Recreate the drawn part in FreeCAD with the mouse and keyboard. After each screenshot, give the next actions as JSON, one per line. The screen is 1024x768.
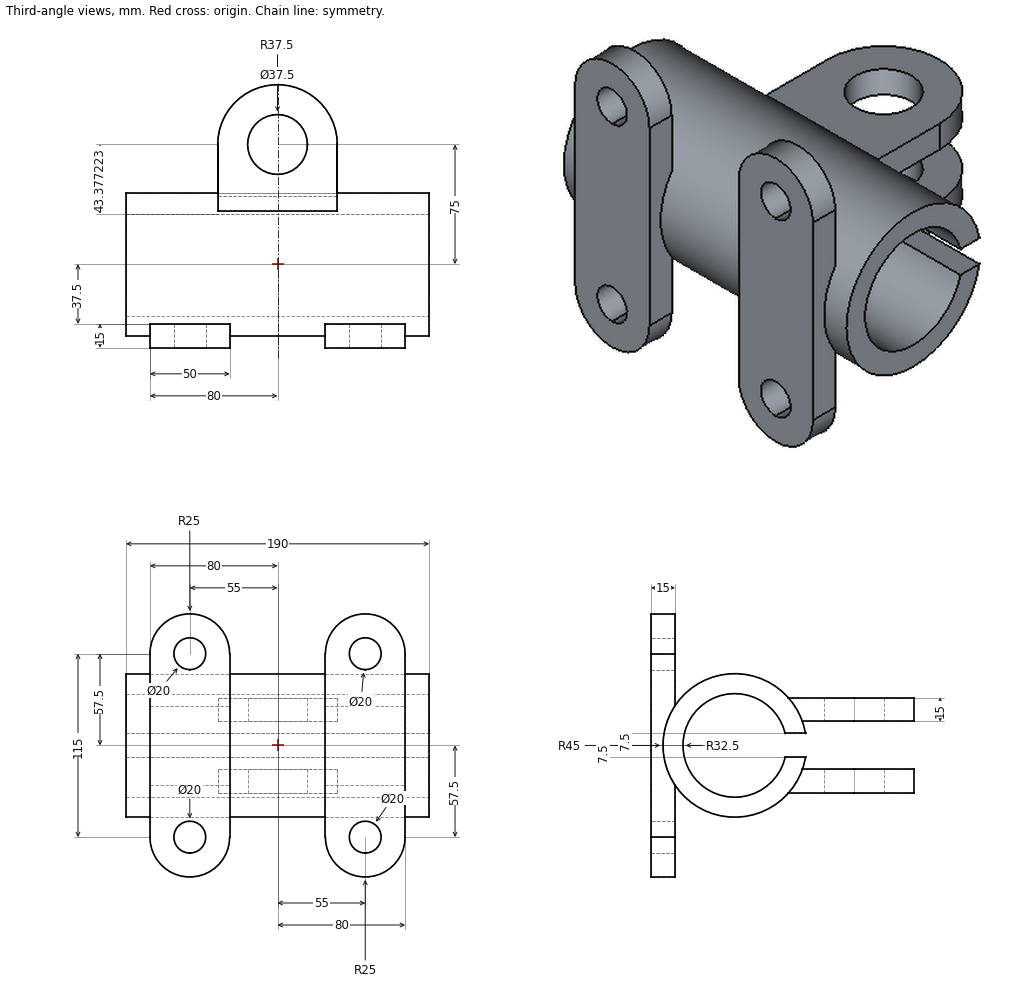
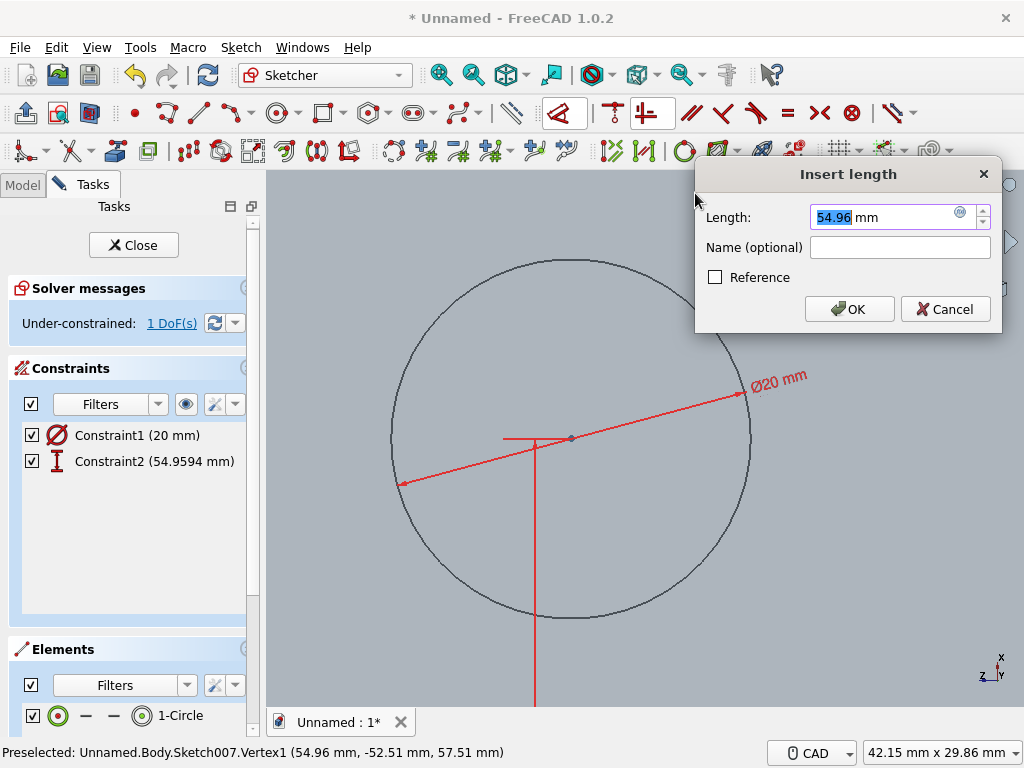
{"action": "type", "text": "55"}
{"action": "key", "text": "Return"}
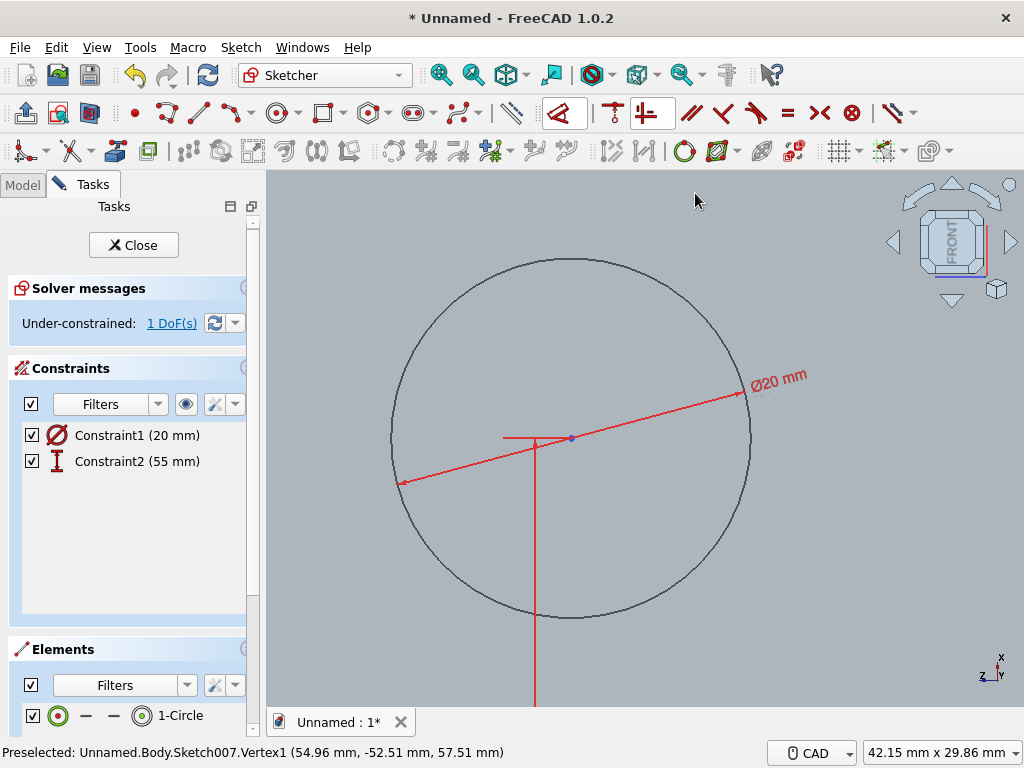
{"action": "left_click", "coordinate": [571, 438]}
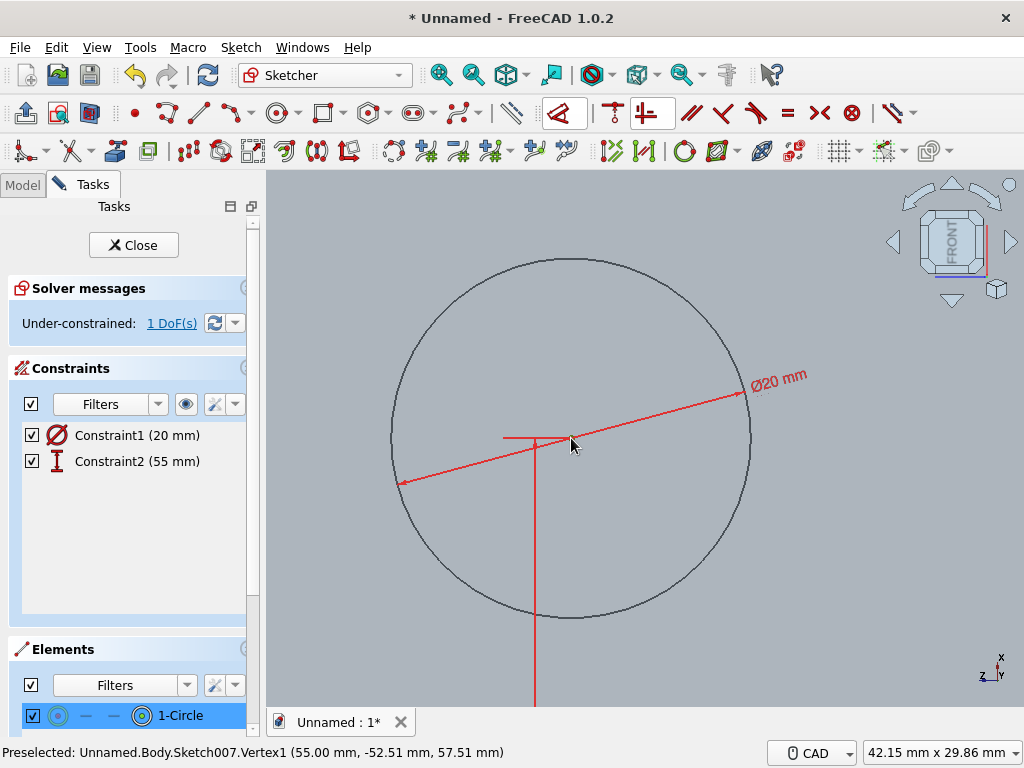
{"action": "left_click", "coordinate": [582, 114]}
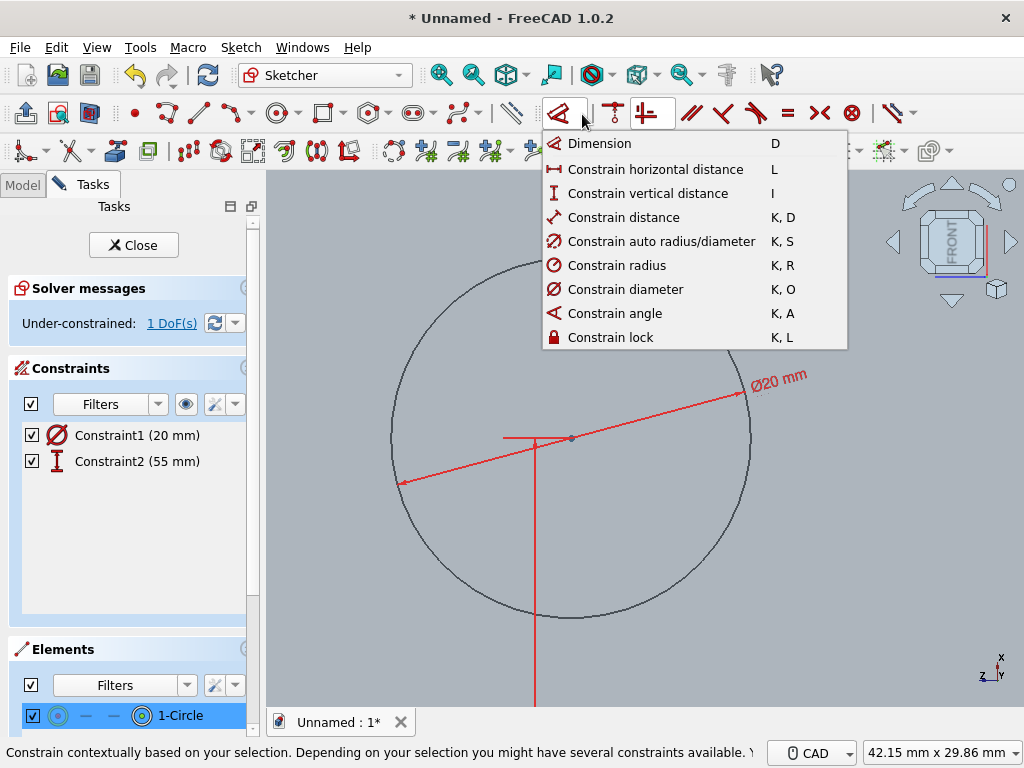
{"action": "left_click", "coordinate": [695, 169]}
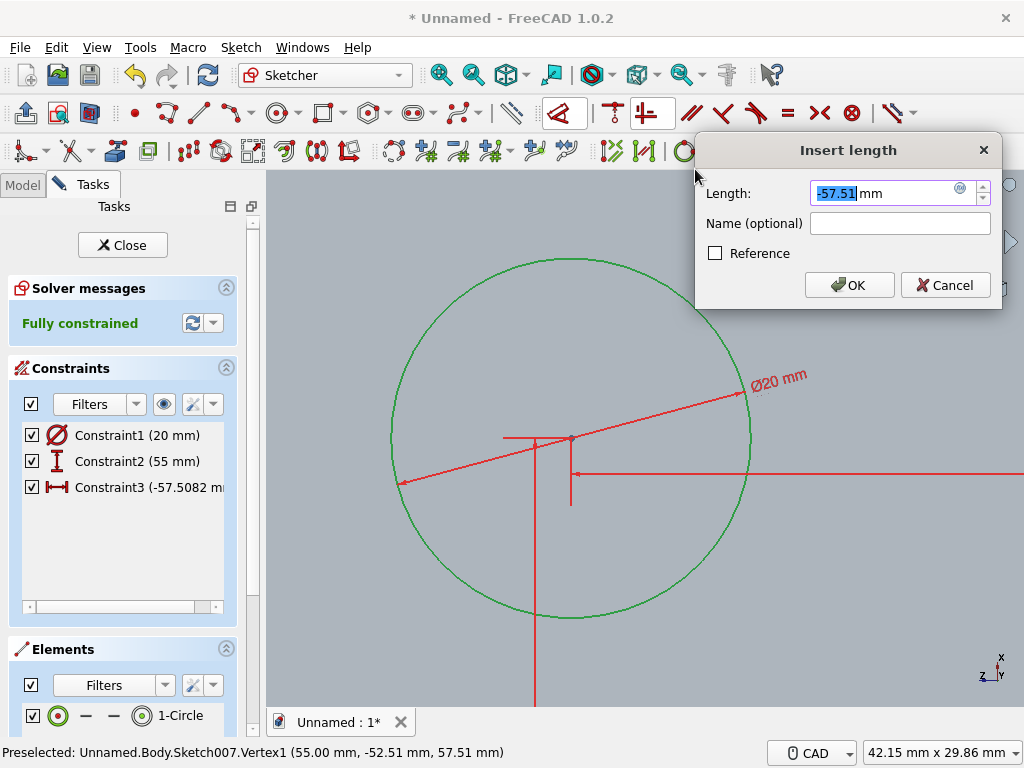
{"action": "type", "text": "-57.5"}
{"action": "key", "text": "Return"}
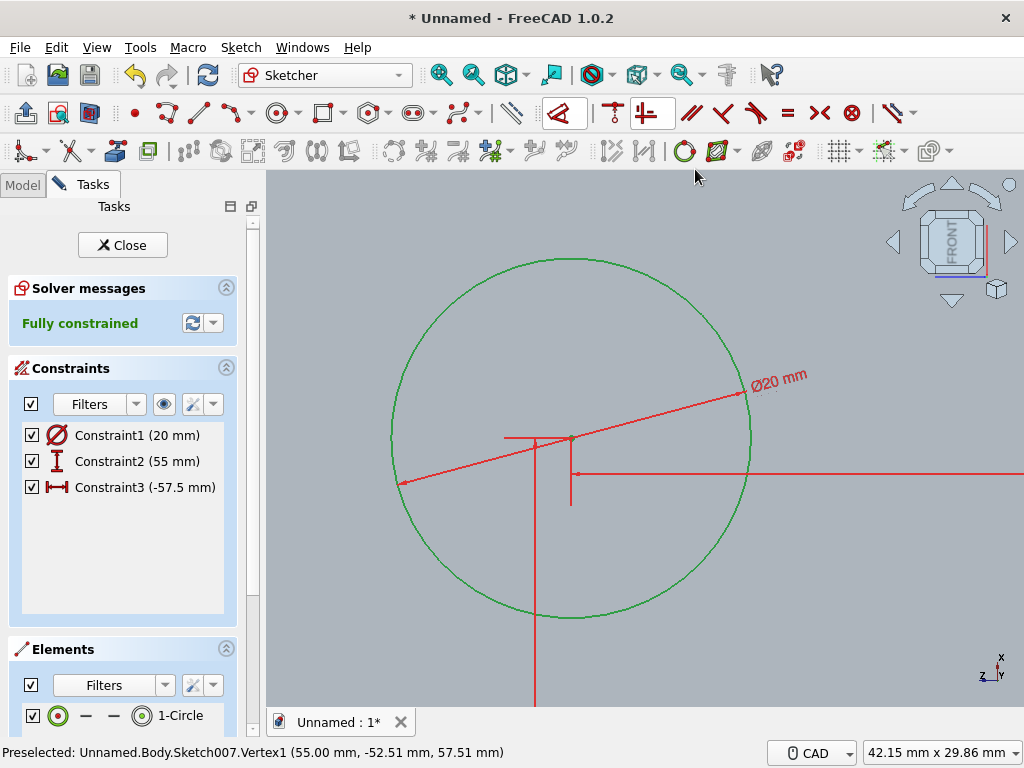
{"action": "left_click", "coordinate": [123, 245]}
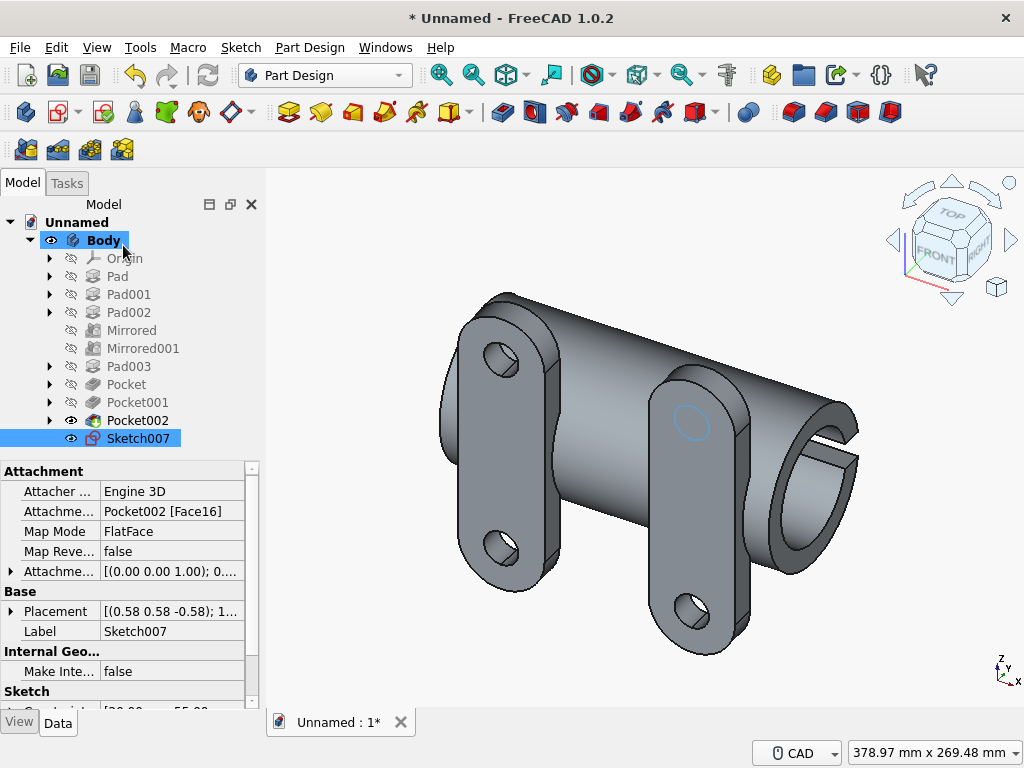
{"action": "left_click", "coordinate": [504, 112]}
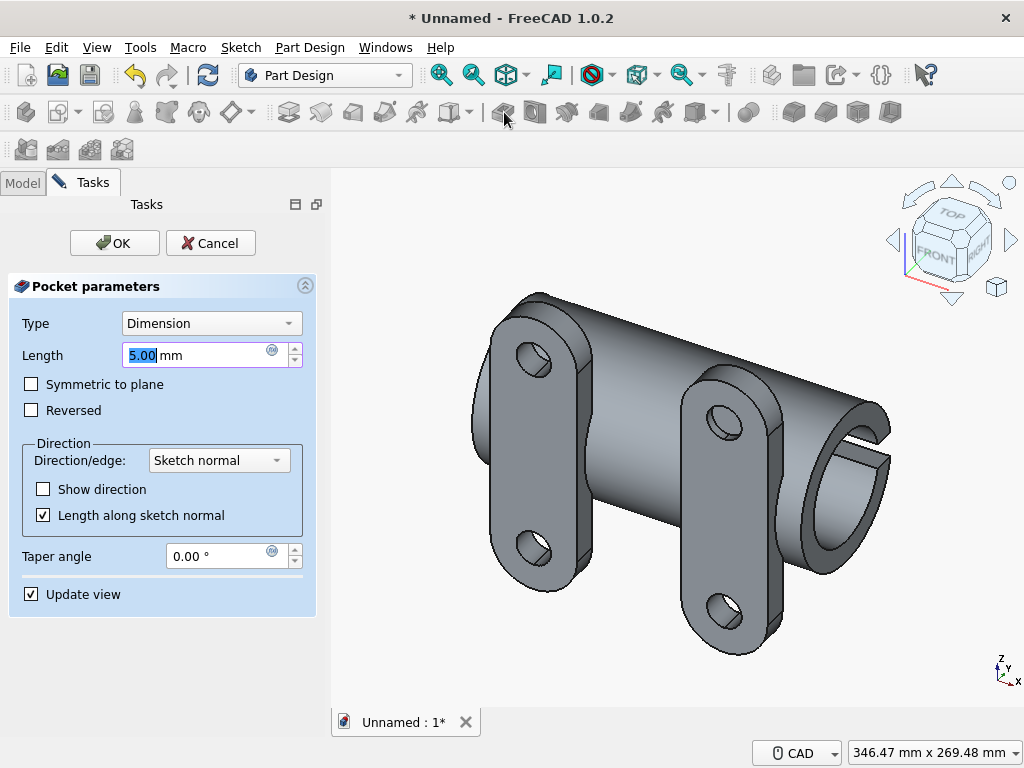
{"action": "left_click", "coordinate": [212, 324]}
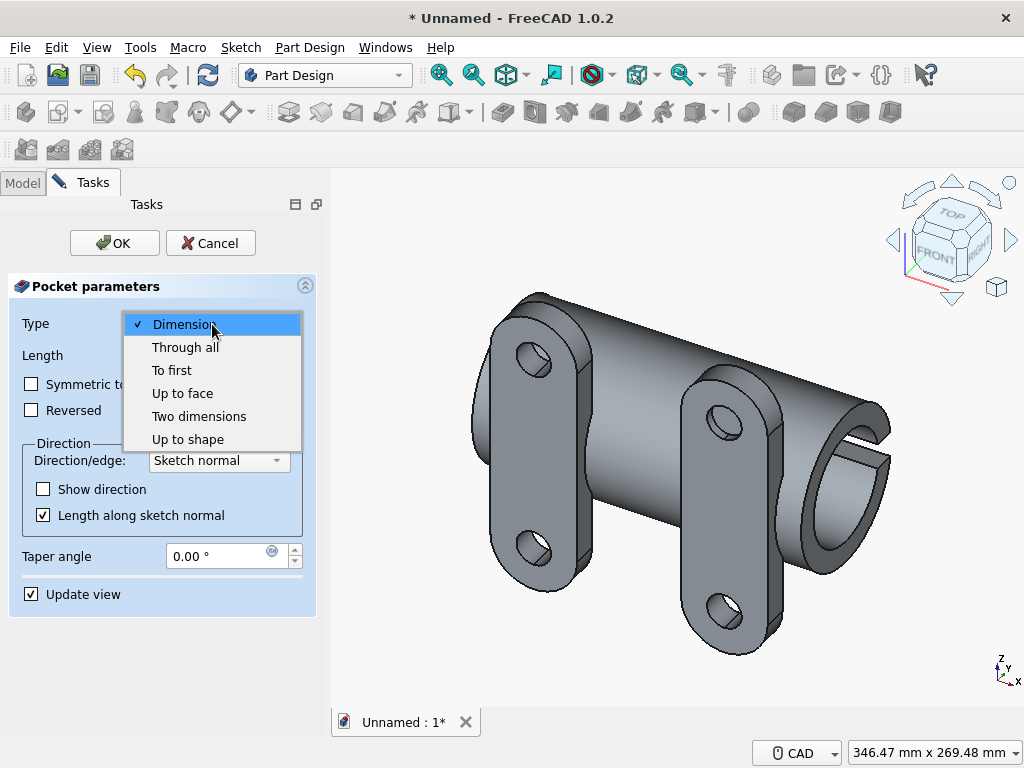
{"action": "left_click", "coordinate": [212, 370]}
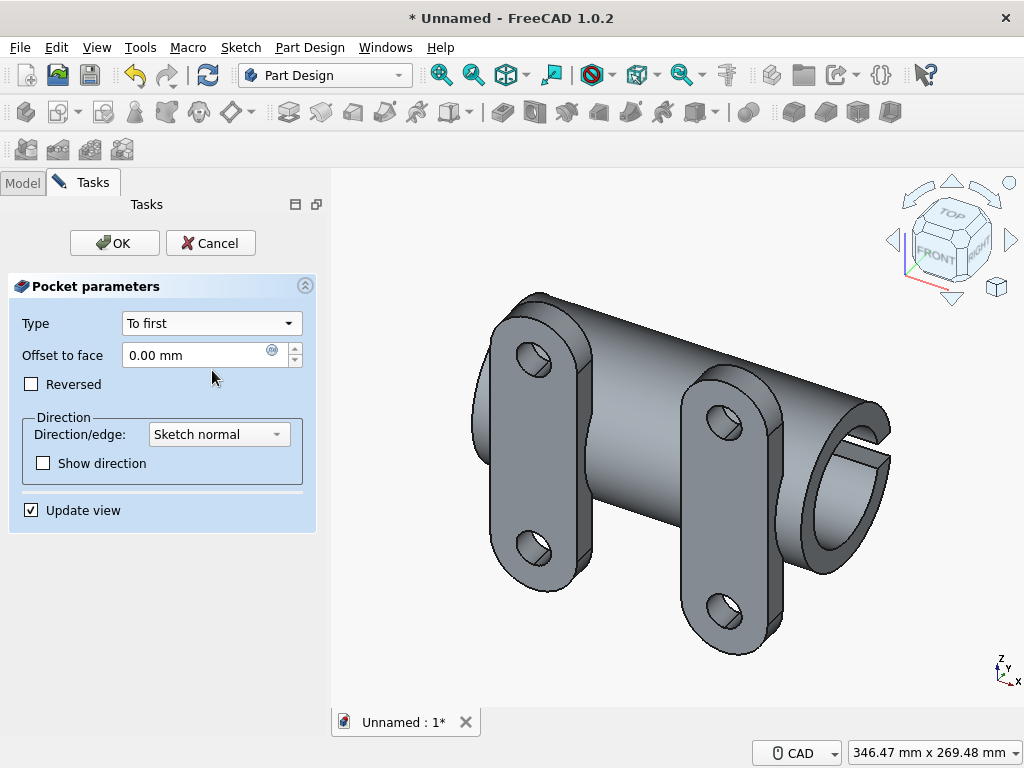
{"action": "left_click", "coordinate": [115, 243]}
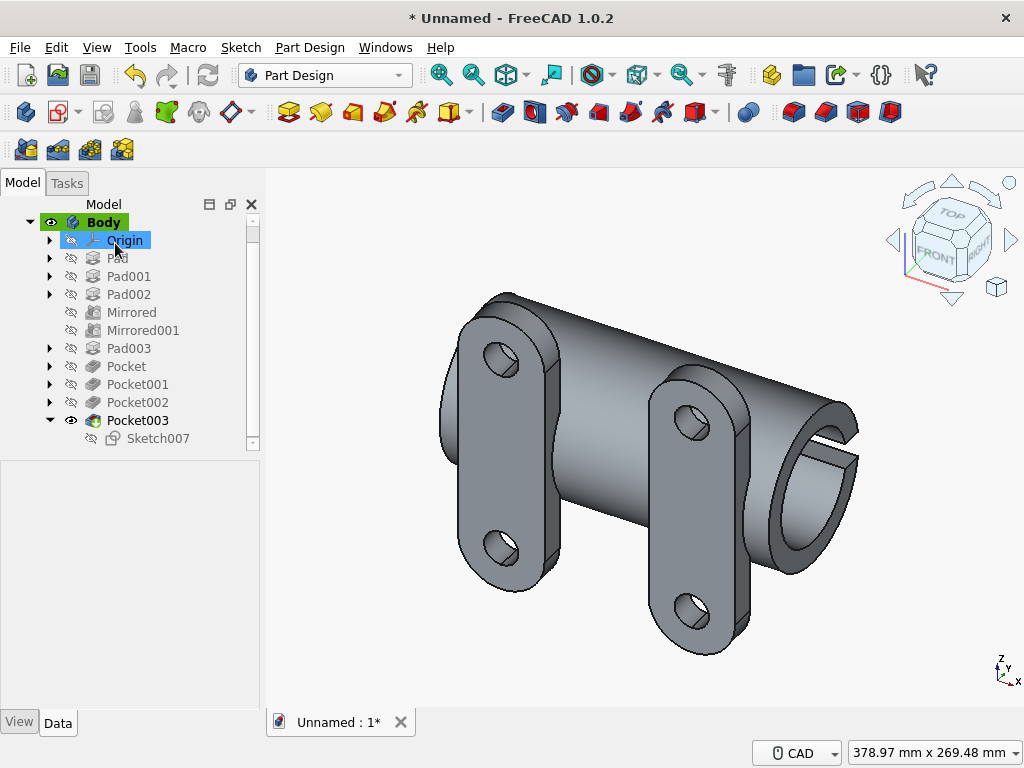
{"action": "left_click", "coordinate": [50, 240]}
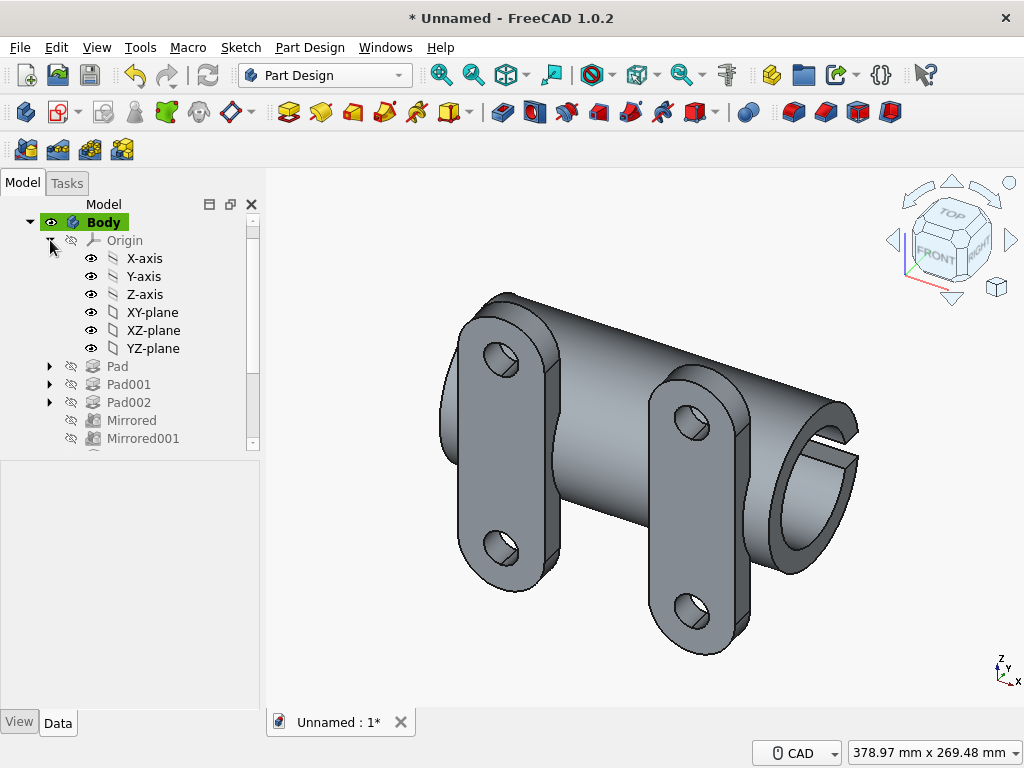
{"action": "left_click", "coordinate": [136, 312]}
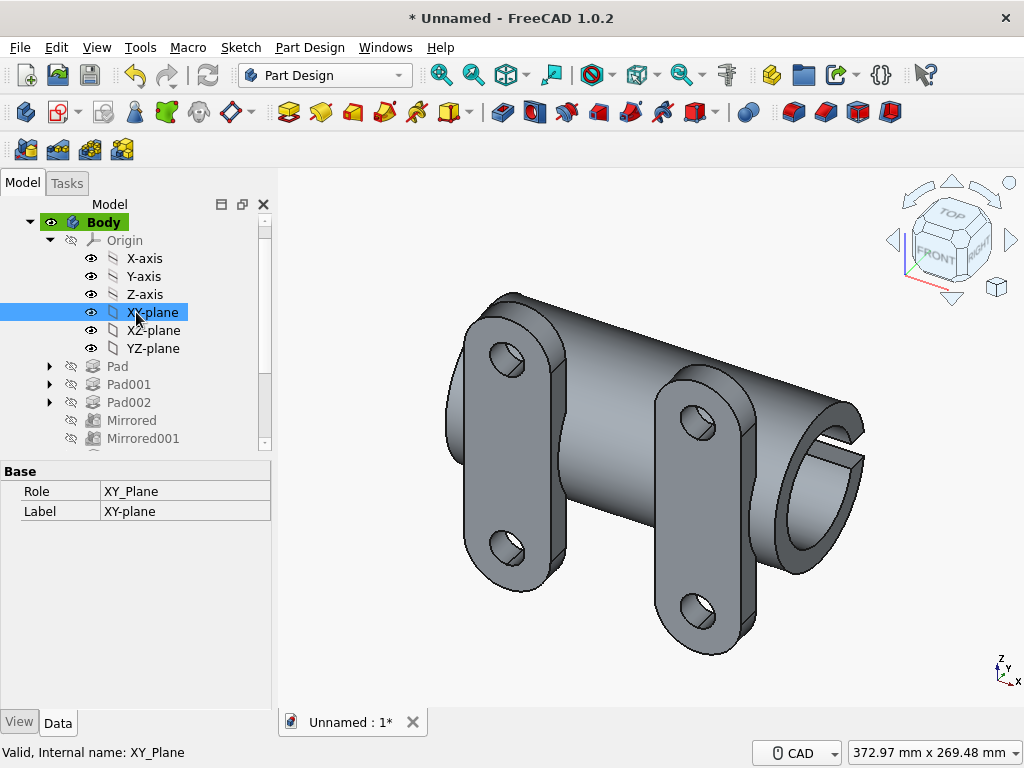
{"action": "left_click", "coordinate": [232, 112]}